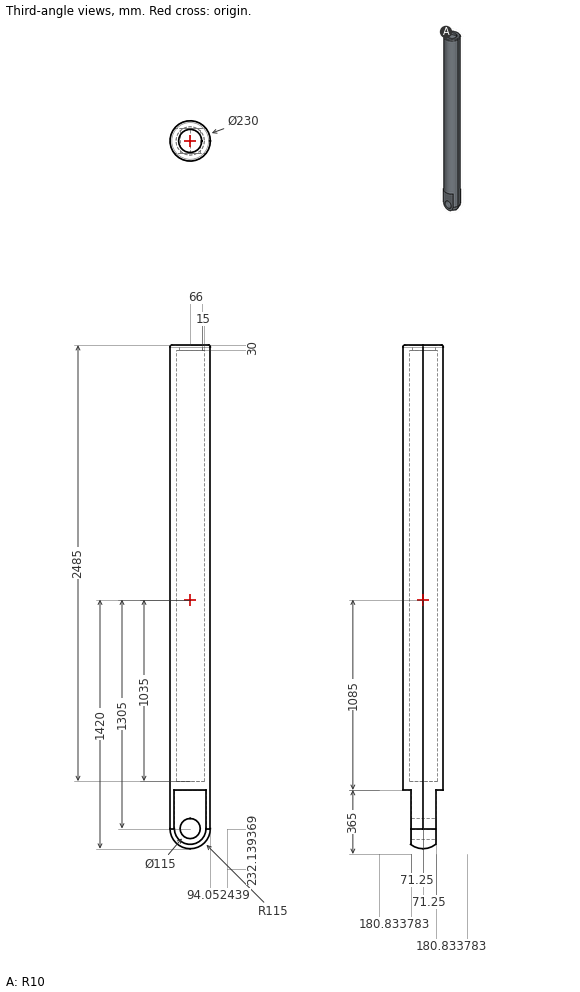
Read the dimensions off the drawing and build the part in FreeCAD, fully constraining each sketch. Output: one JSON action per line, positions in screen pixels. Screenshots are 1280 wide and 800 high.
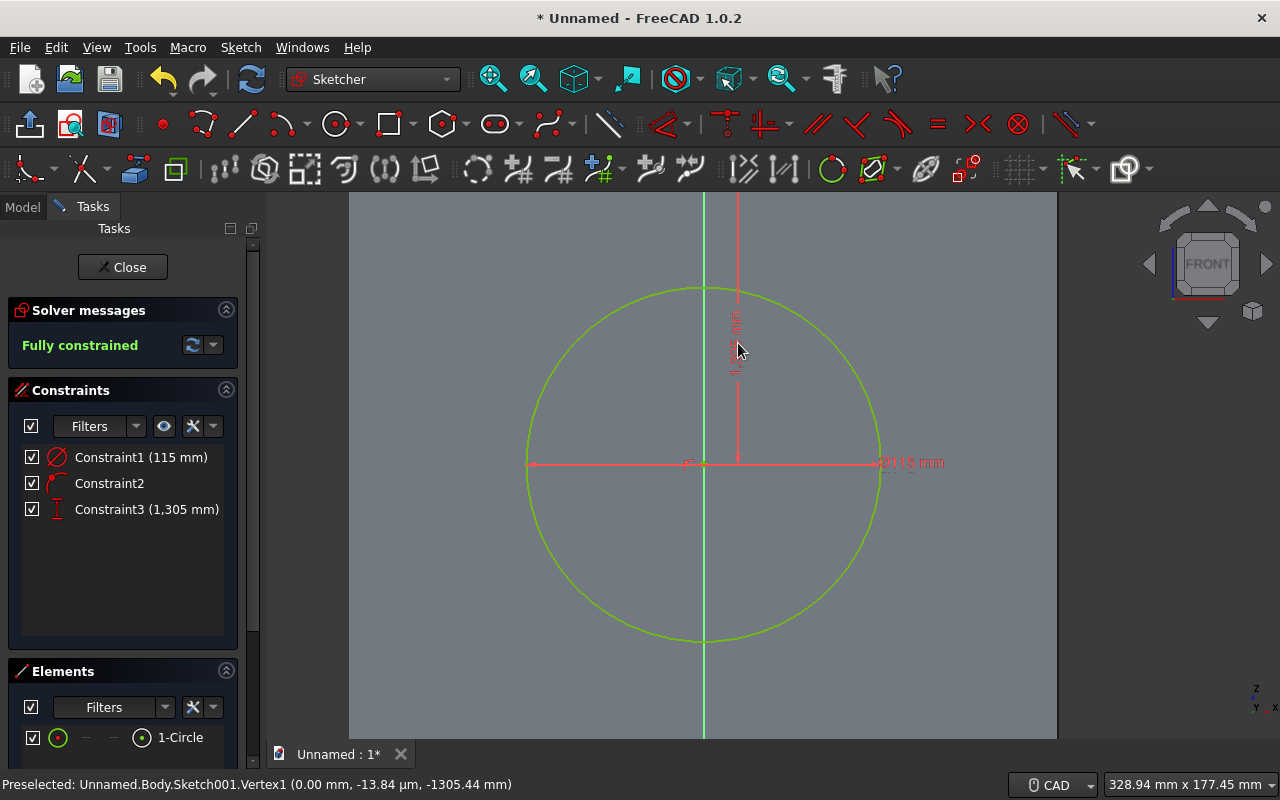
{"action": "left_click", "coordinate": [123, 267]}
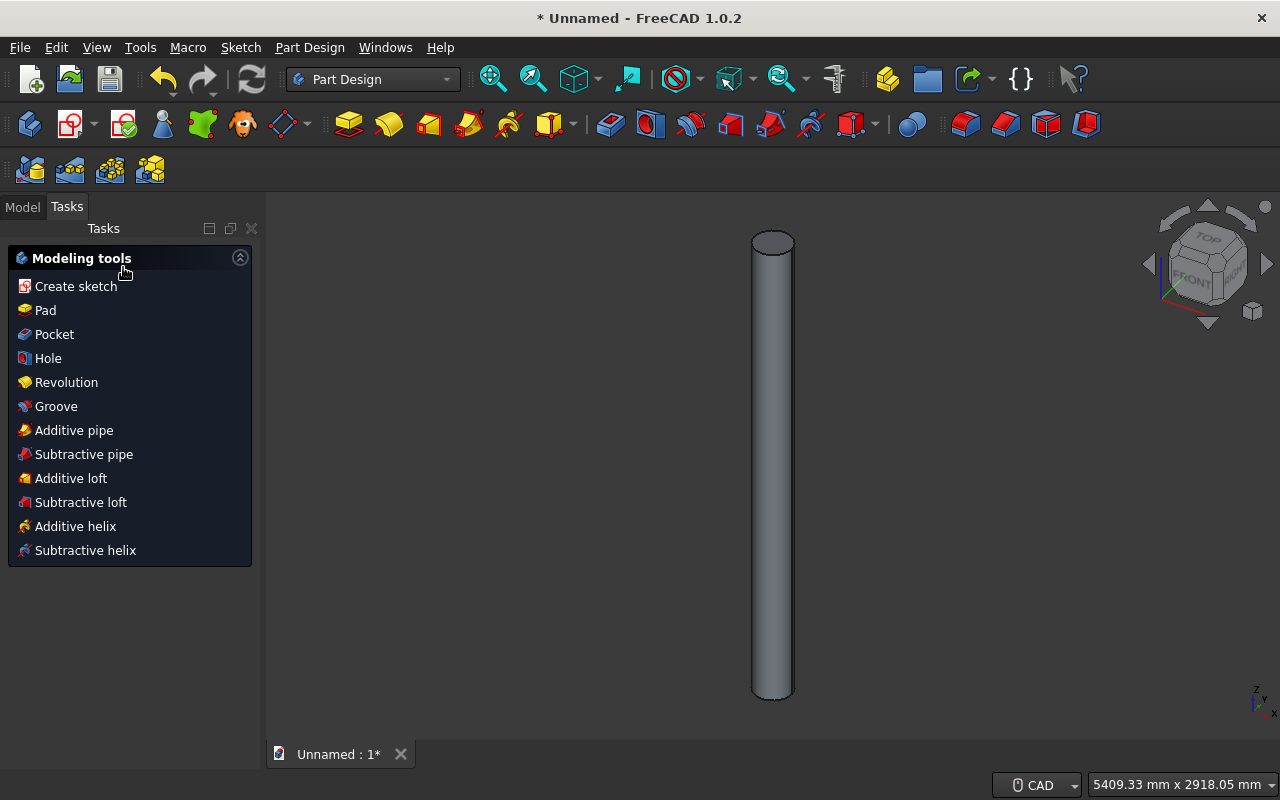
{"action": "left_click", "coordinate": [612, 124]}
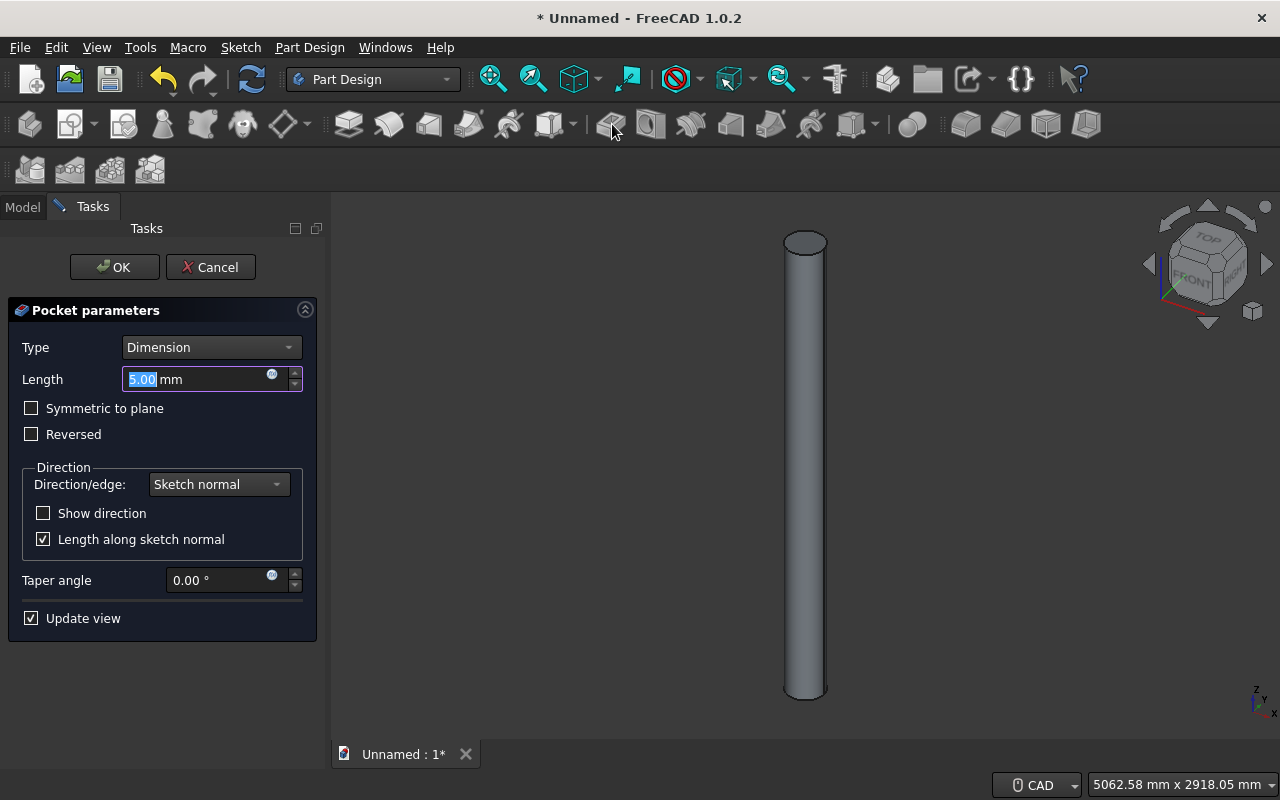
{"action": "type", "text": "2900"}
{"action": "key", "text": "Tab"}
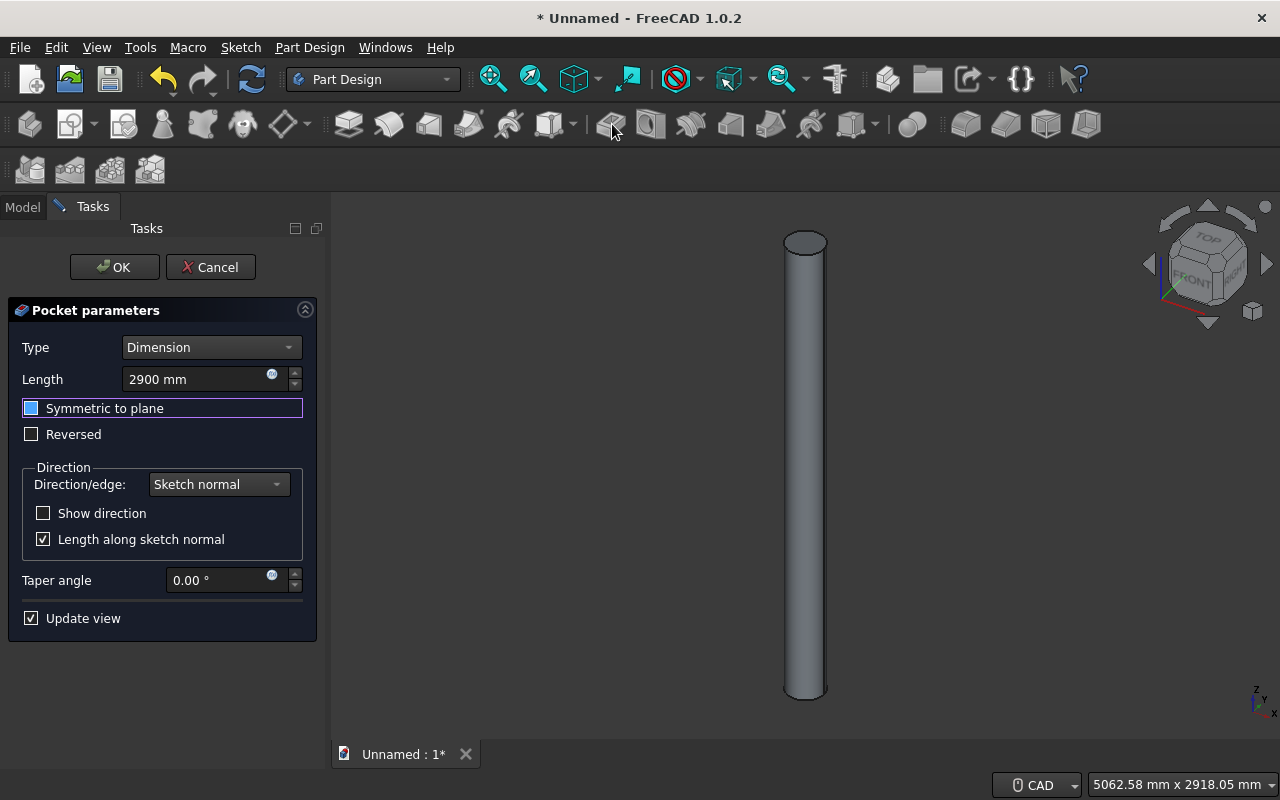
{"action": "left_click", "coordinate": [30, 408]}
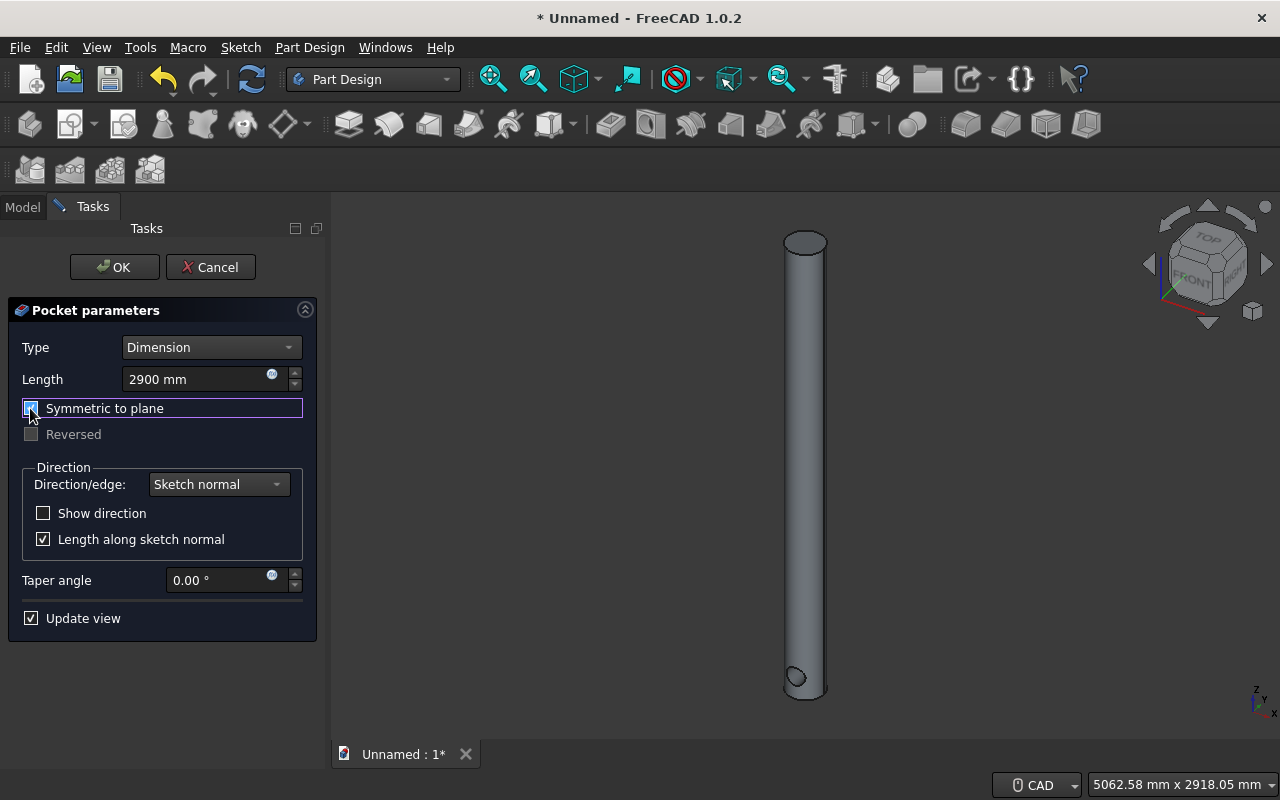
{"action": "left_click", "coordinate": [115, 267]}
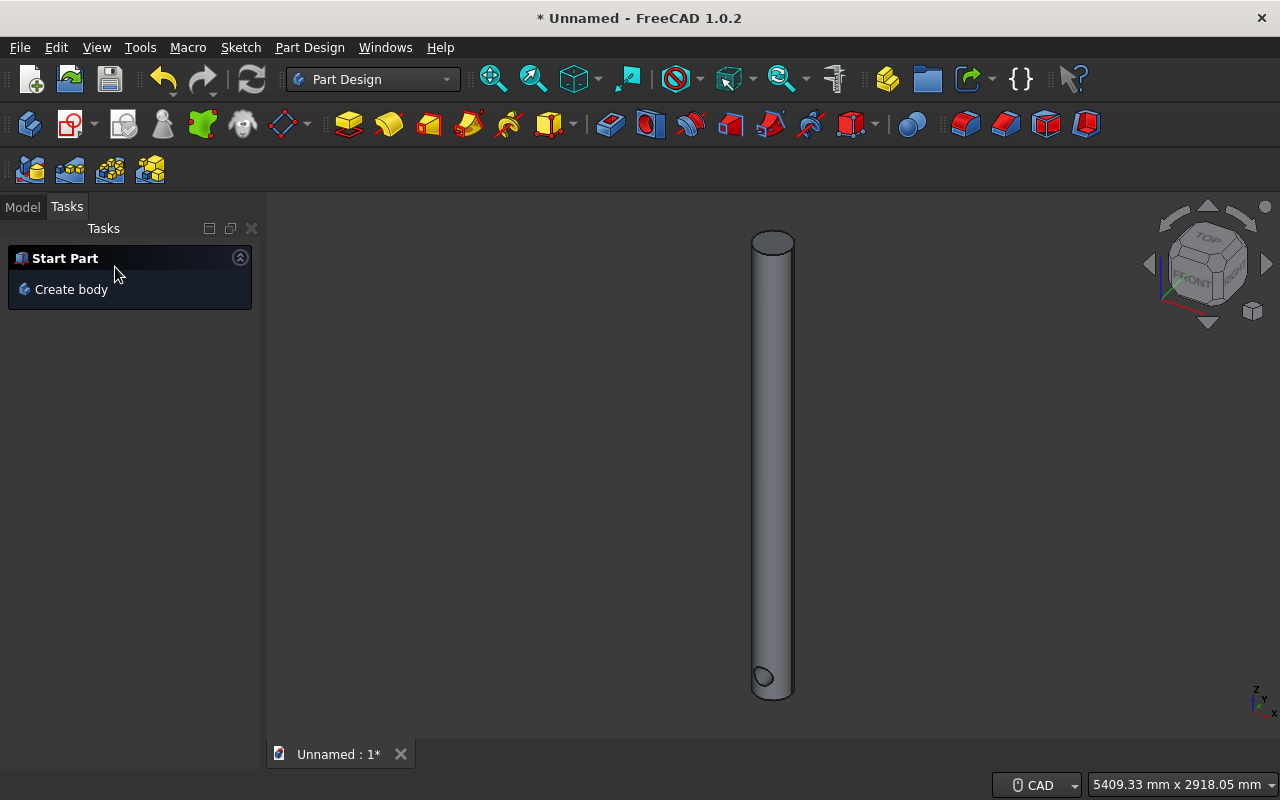
{"action": "left_click", "coordinate": [70, 124]}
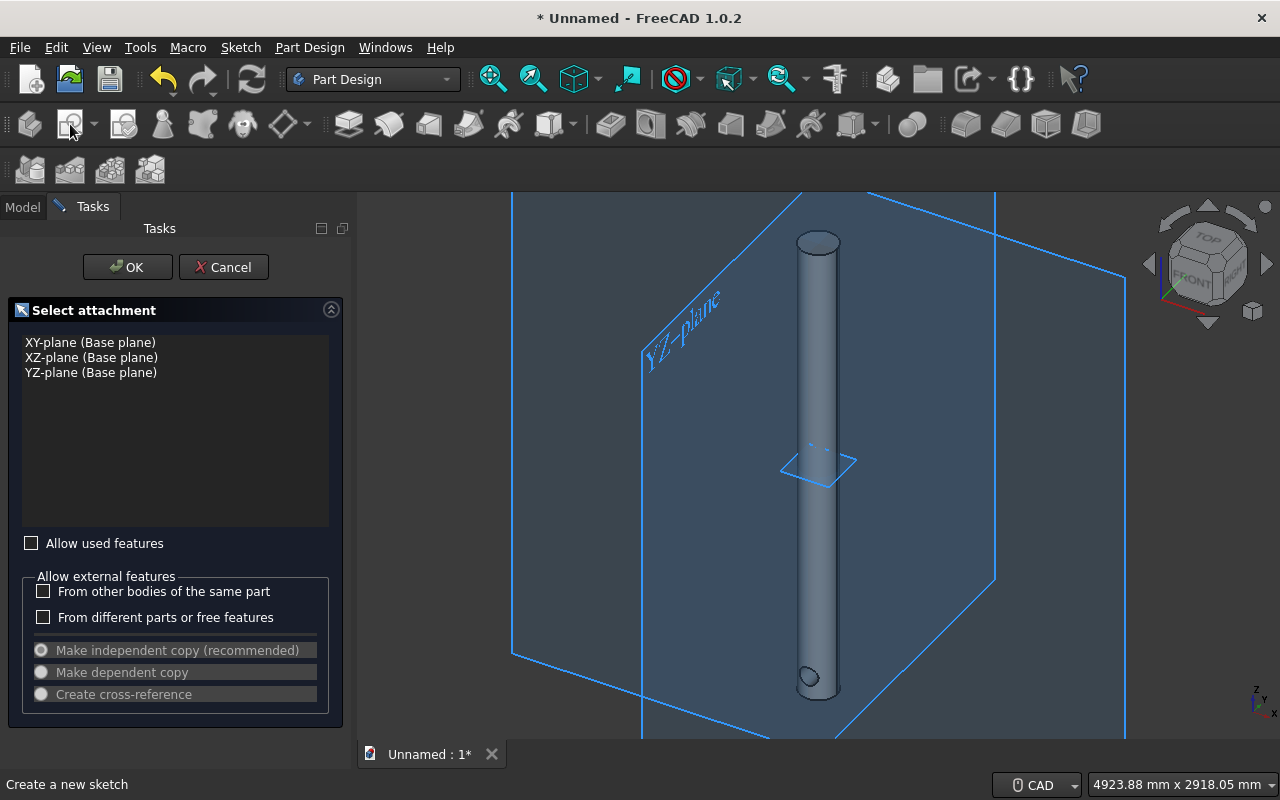
{"action": "left_click", "coordinate": [82, 372]}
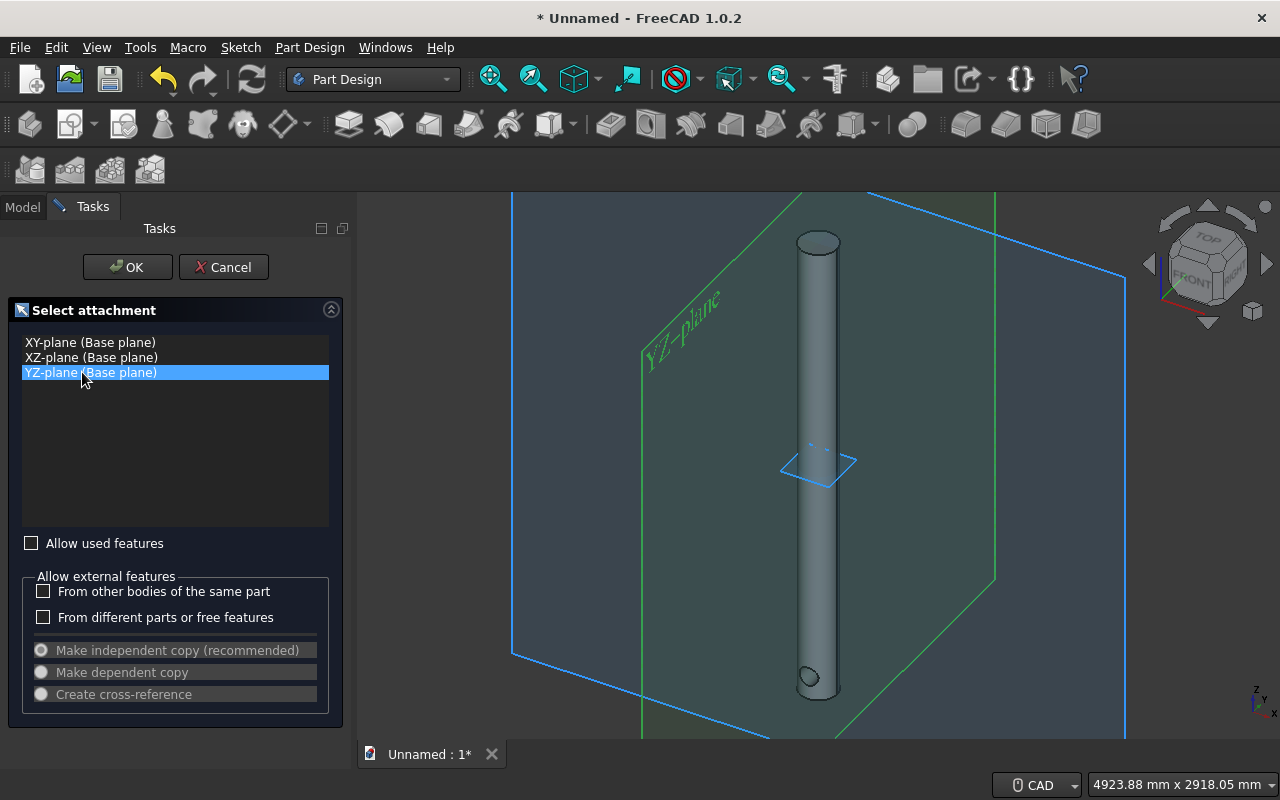
{"action": "left_click", "coordinate": [128, 267]}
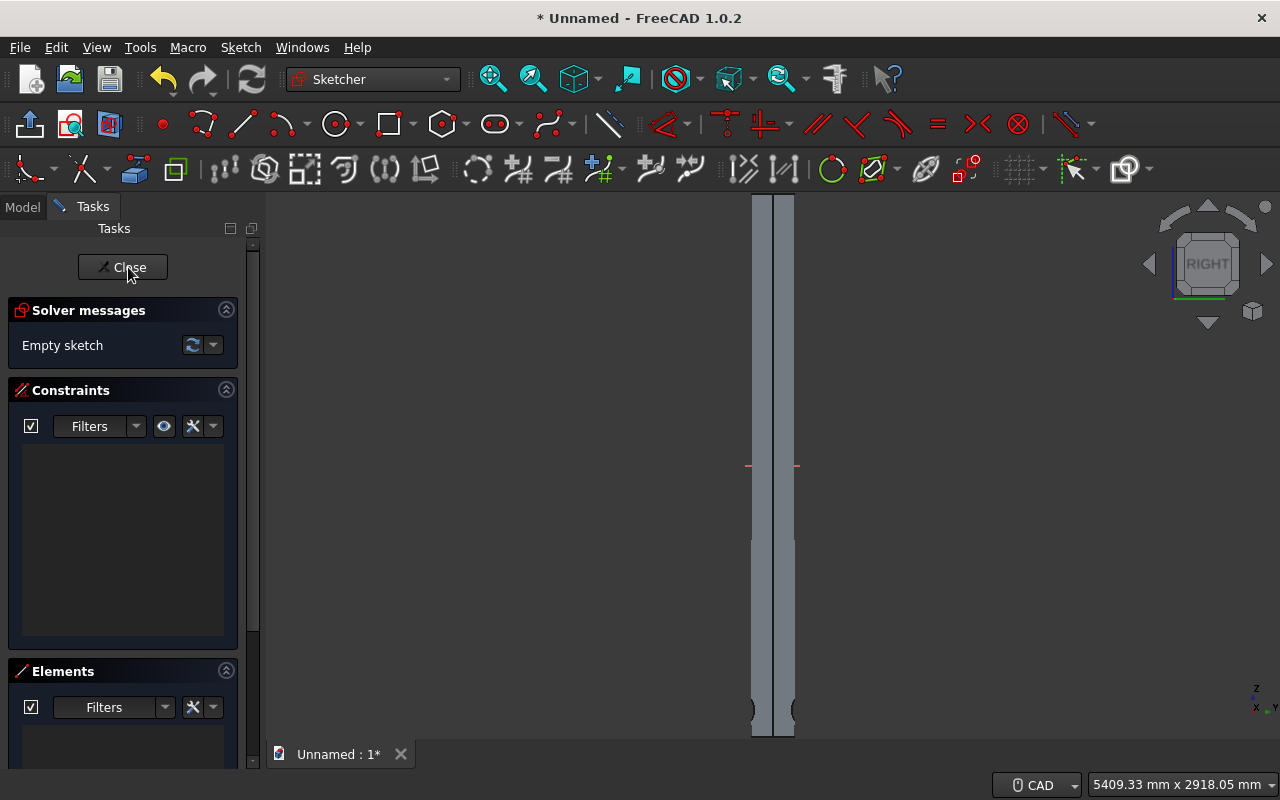
{"action": "key", "text": "q s"}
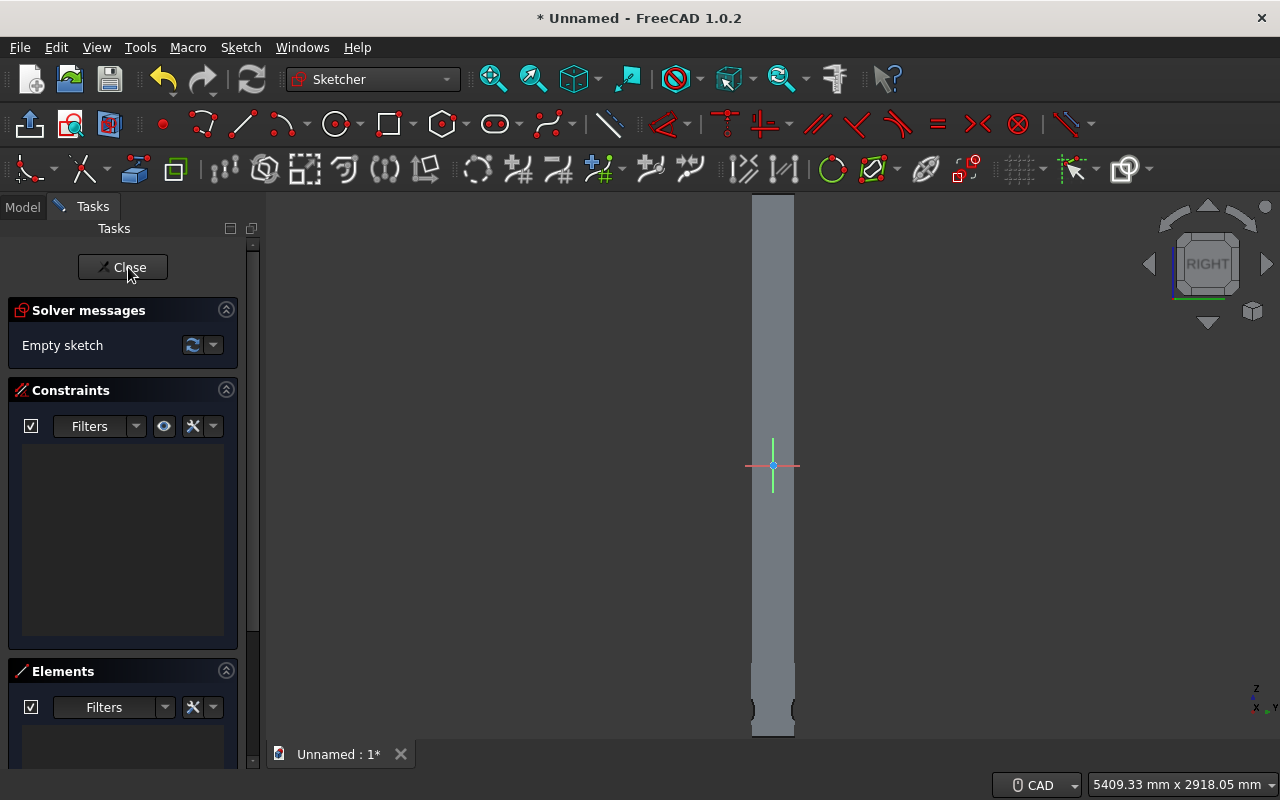
{"action": "scroll", "coordinate": [704, 466], "scroll_direction": "down", "scroll_amount": 5}